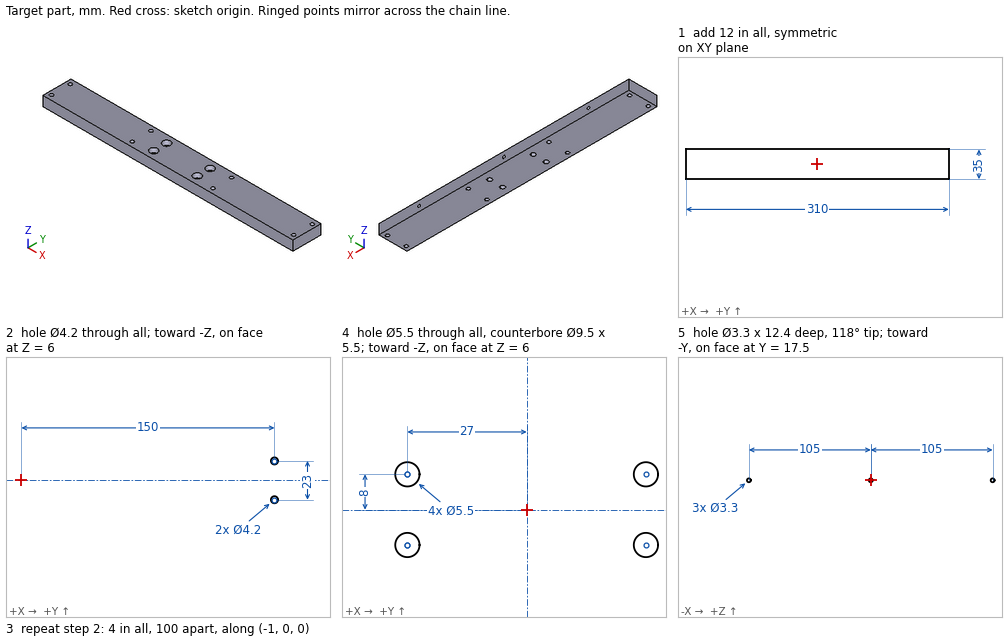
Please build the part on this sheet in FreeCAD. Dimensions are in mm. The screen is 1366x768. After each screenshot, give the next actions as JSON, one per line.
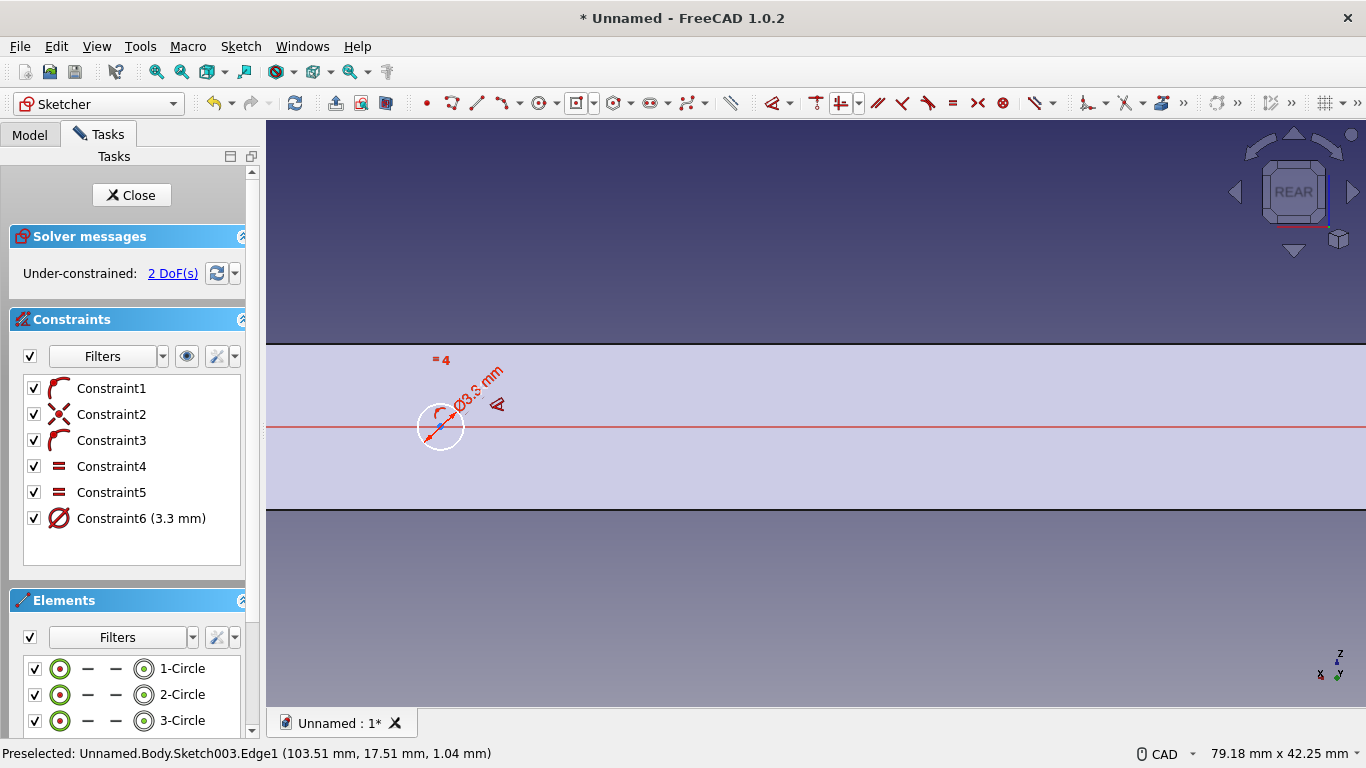
{"action": "scroll", "coordinate": [456, 410], "scroll_direction": "down", "scroll_amount": 8}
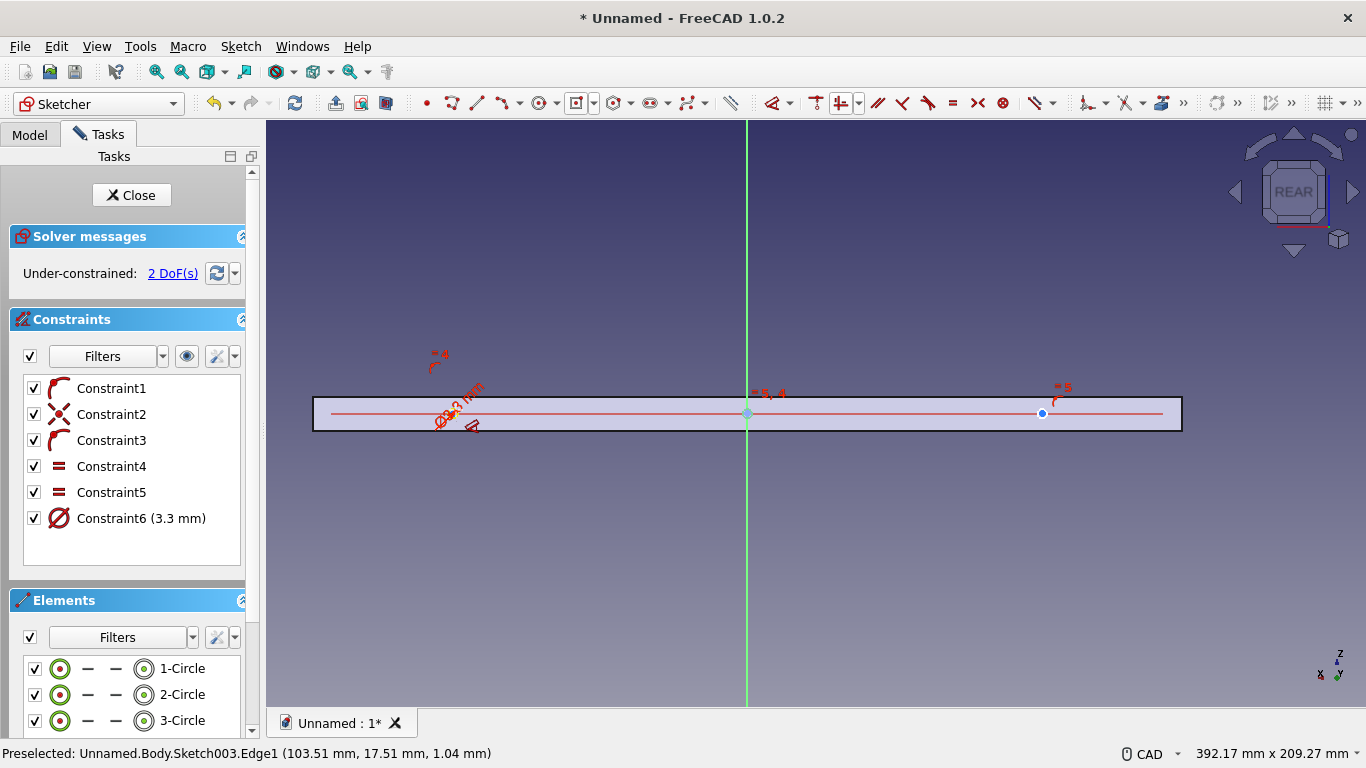
{"action": "left_click", "coordinate": [453, 414]}
{"action": "left_click", "coordinate": [600, 448]}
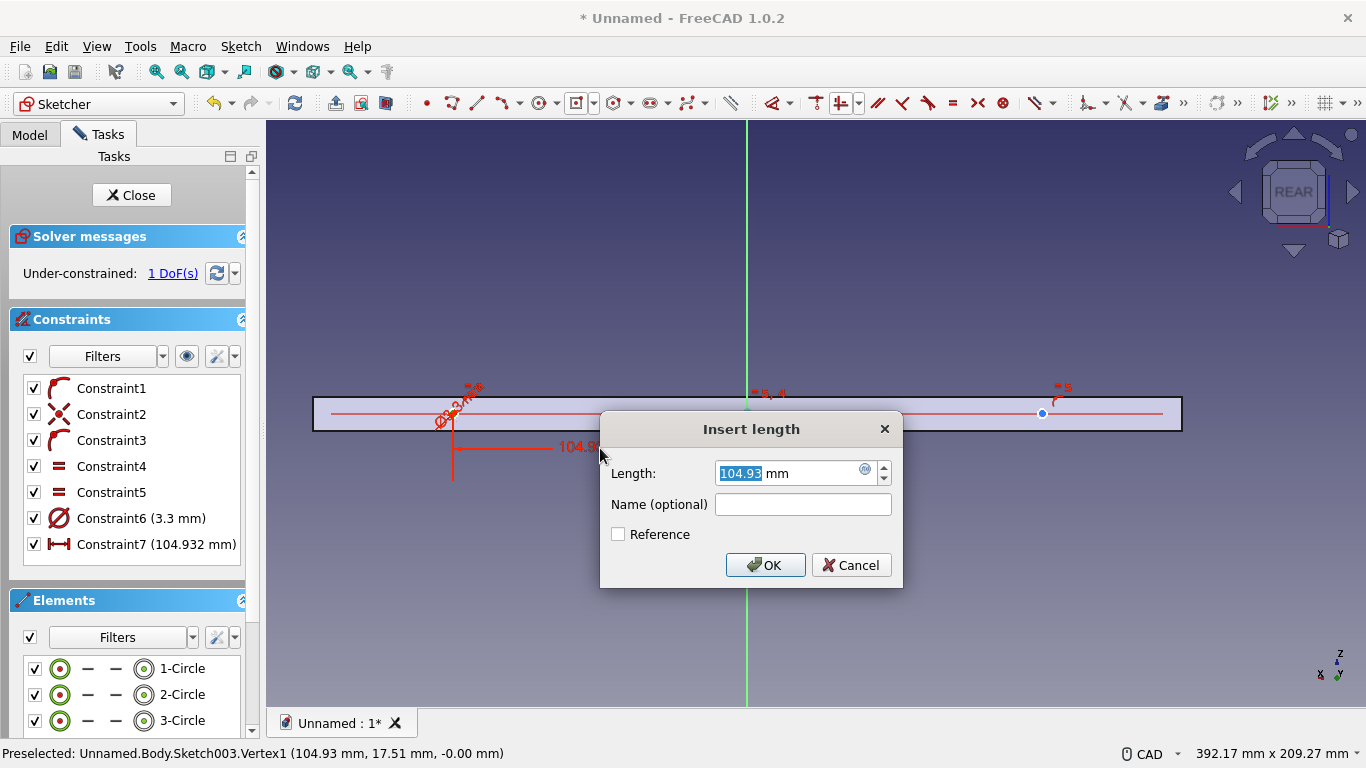
{"action": "type", "text": "105"}
{"action": "key", "text": "Return"}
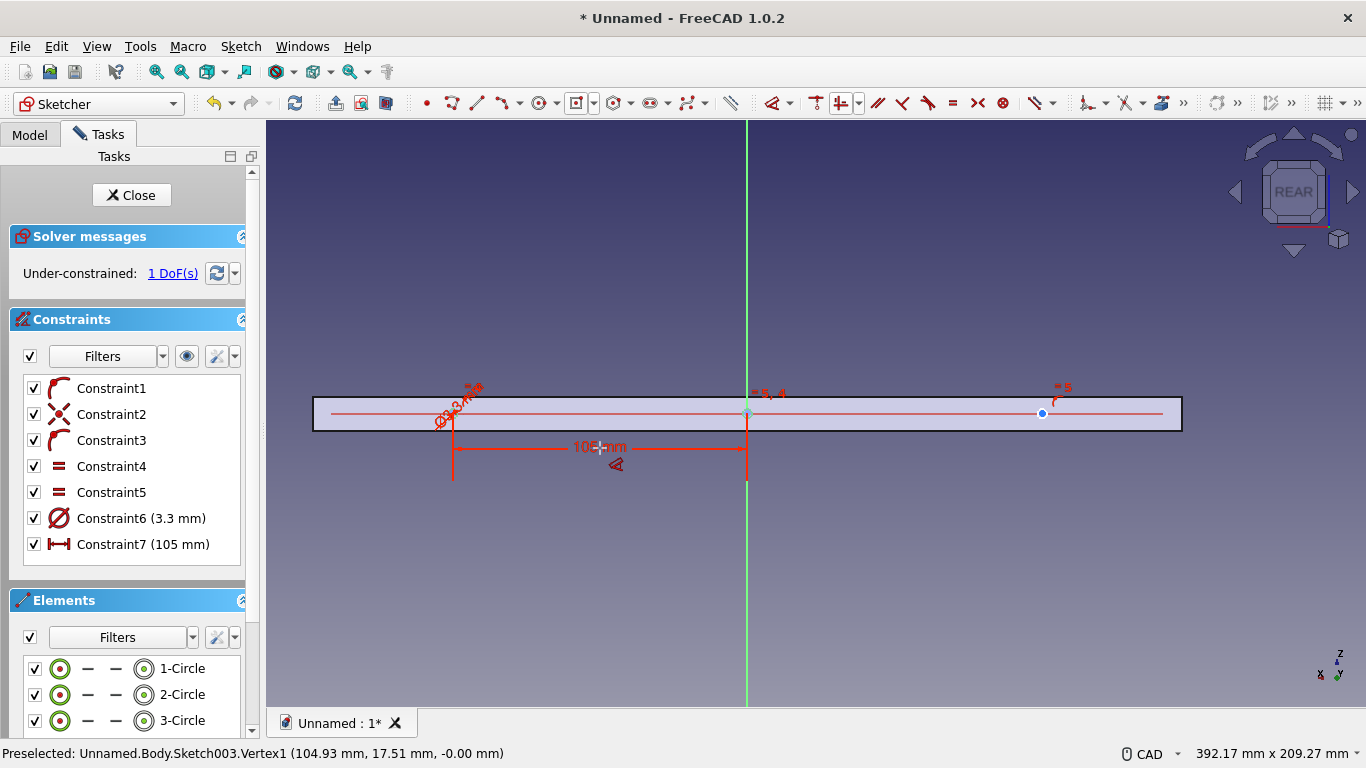
{"action": "left_click", "coordinate": [1042, 414]}
{"action": "left_click", "coordinate": [895, 448]}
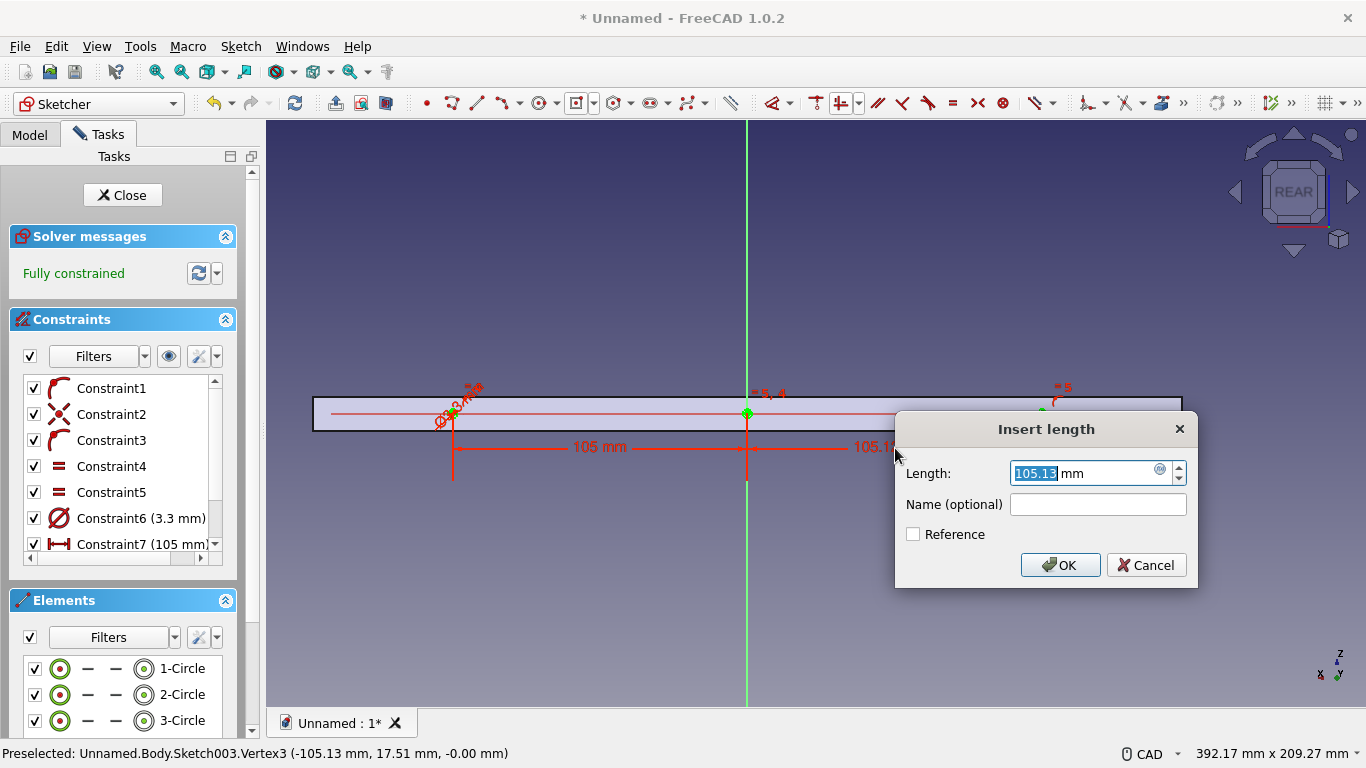
{"action": "type", "text": "105"}
{"action": "key", "text": "Return"}
{"action": "key", "text": "Escape"}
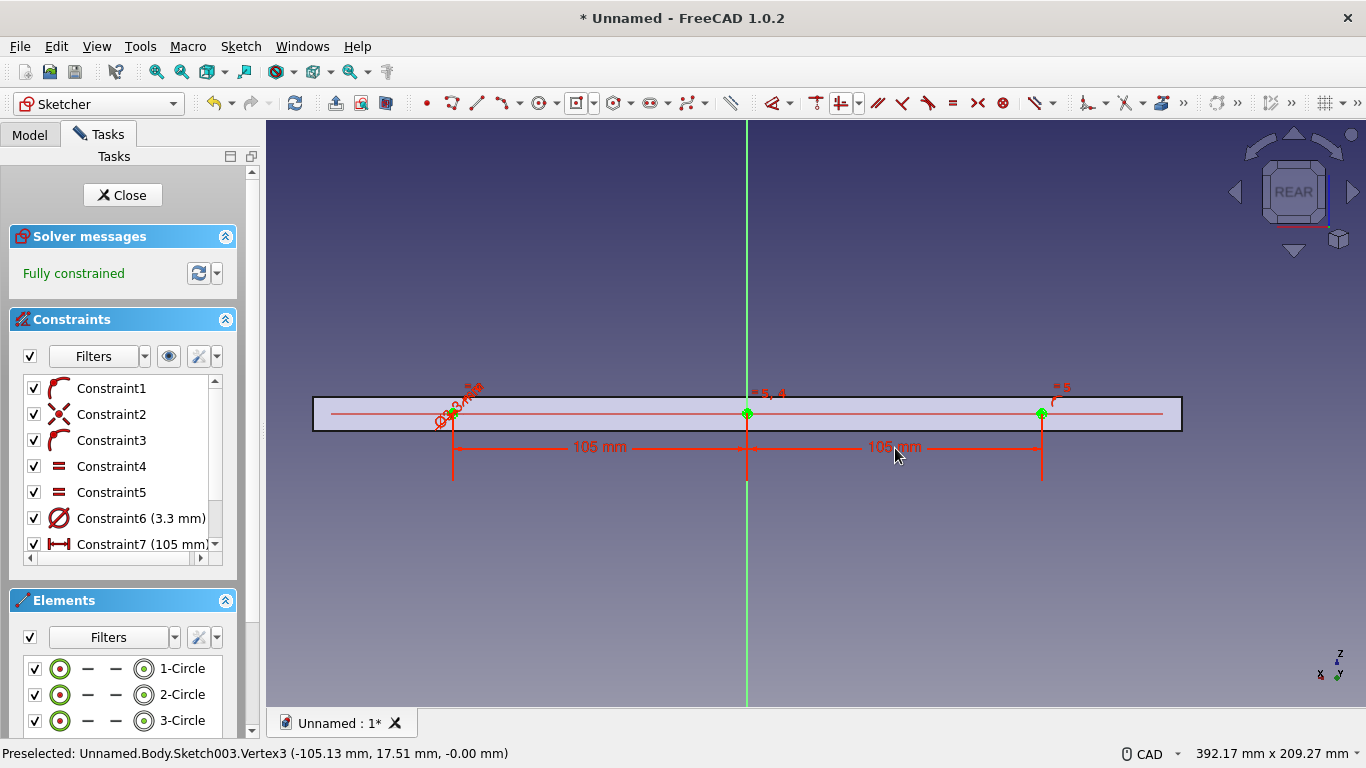
{"action": "left_click", "coordinate": [123, 195]}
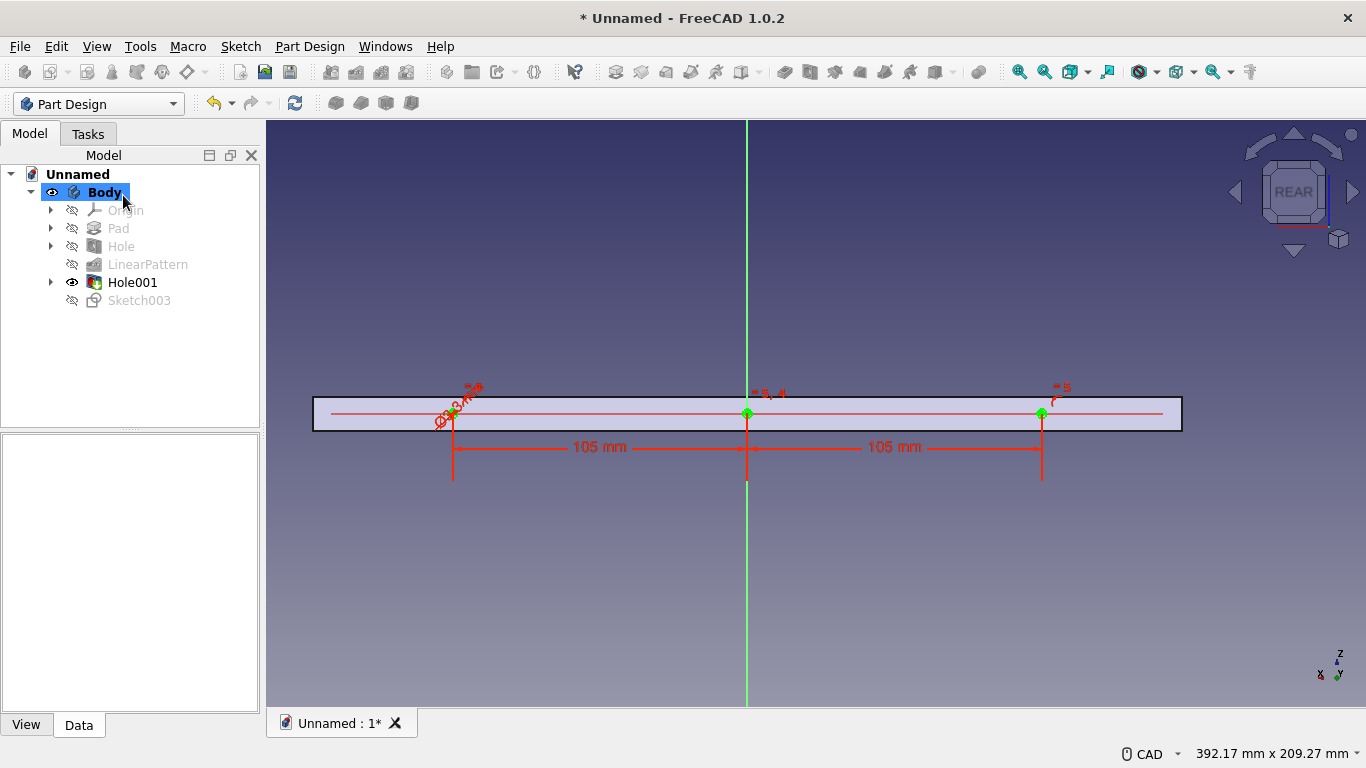
{"action": "left_click", "coordinate": [810, 72]}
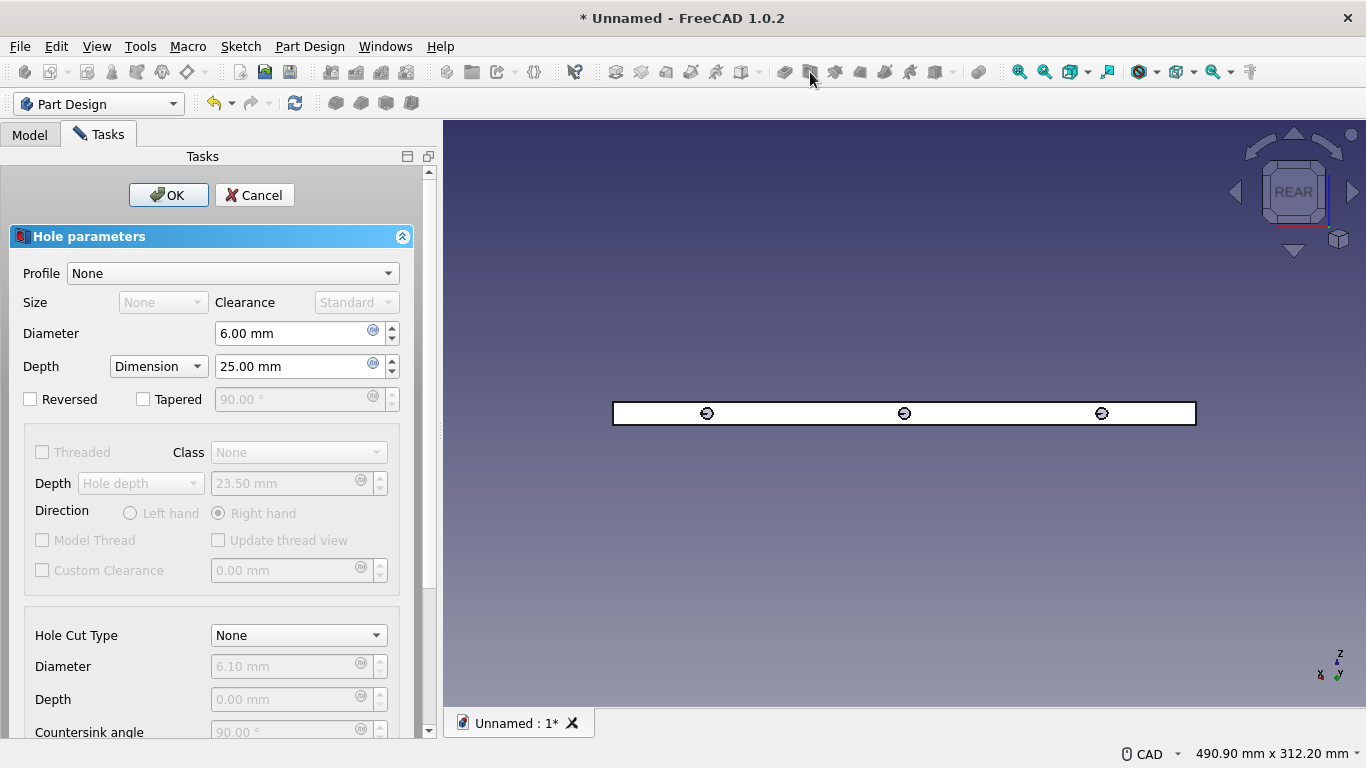
{"action": "triple_click", "coordinate": [300, 334]}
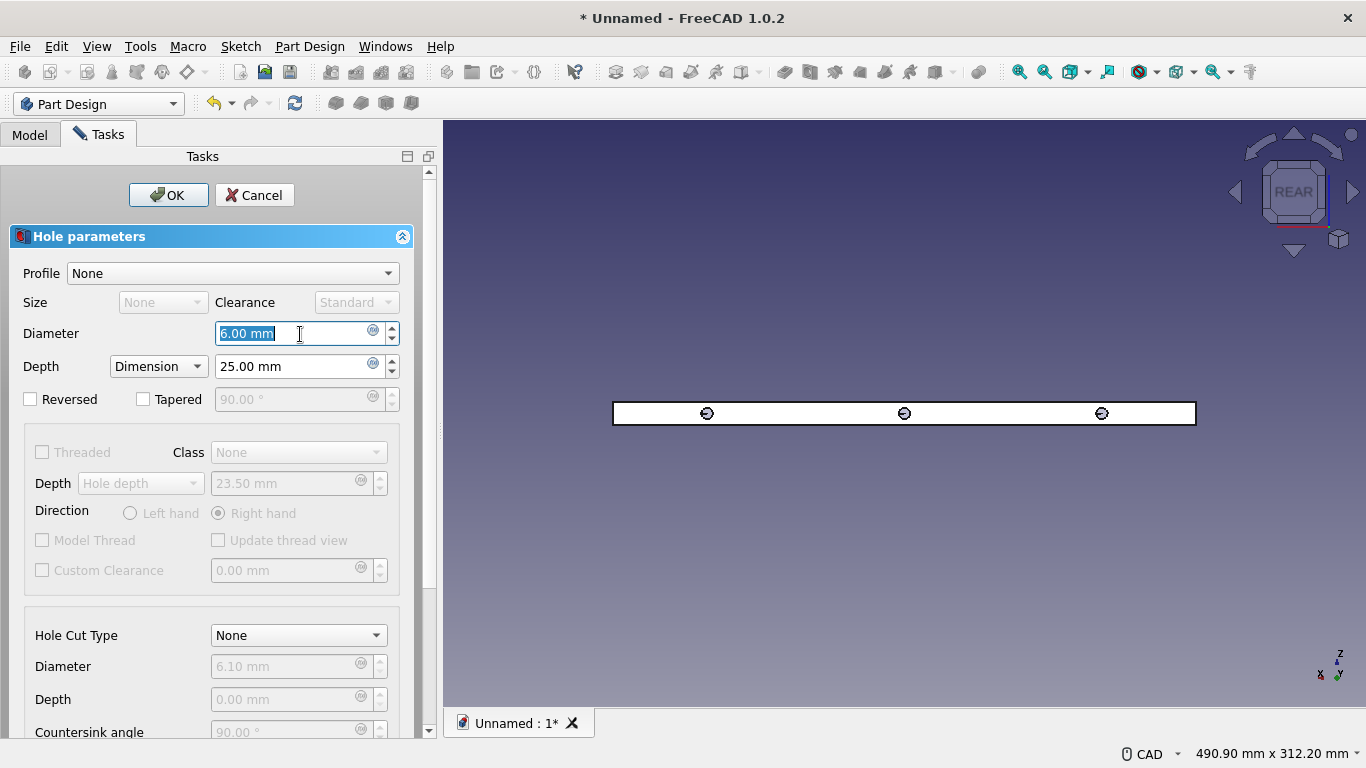
{"action": "type", "text": "3.3"}
{"action": "key", "text": "Tab"}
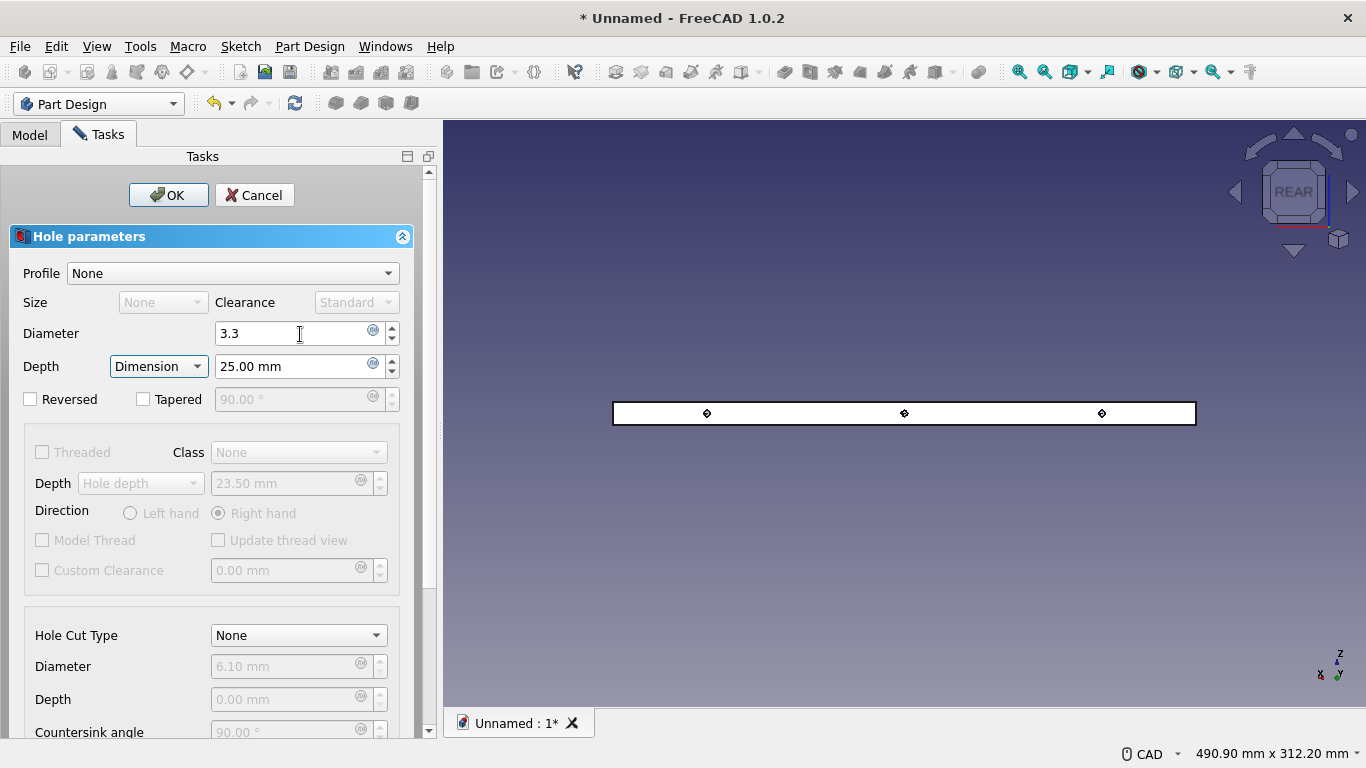
{"action": "triple_click", "coordinate": [300, 366]}